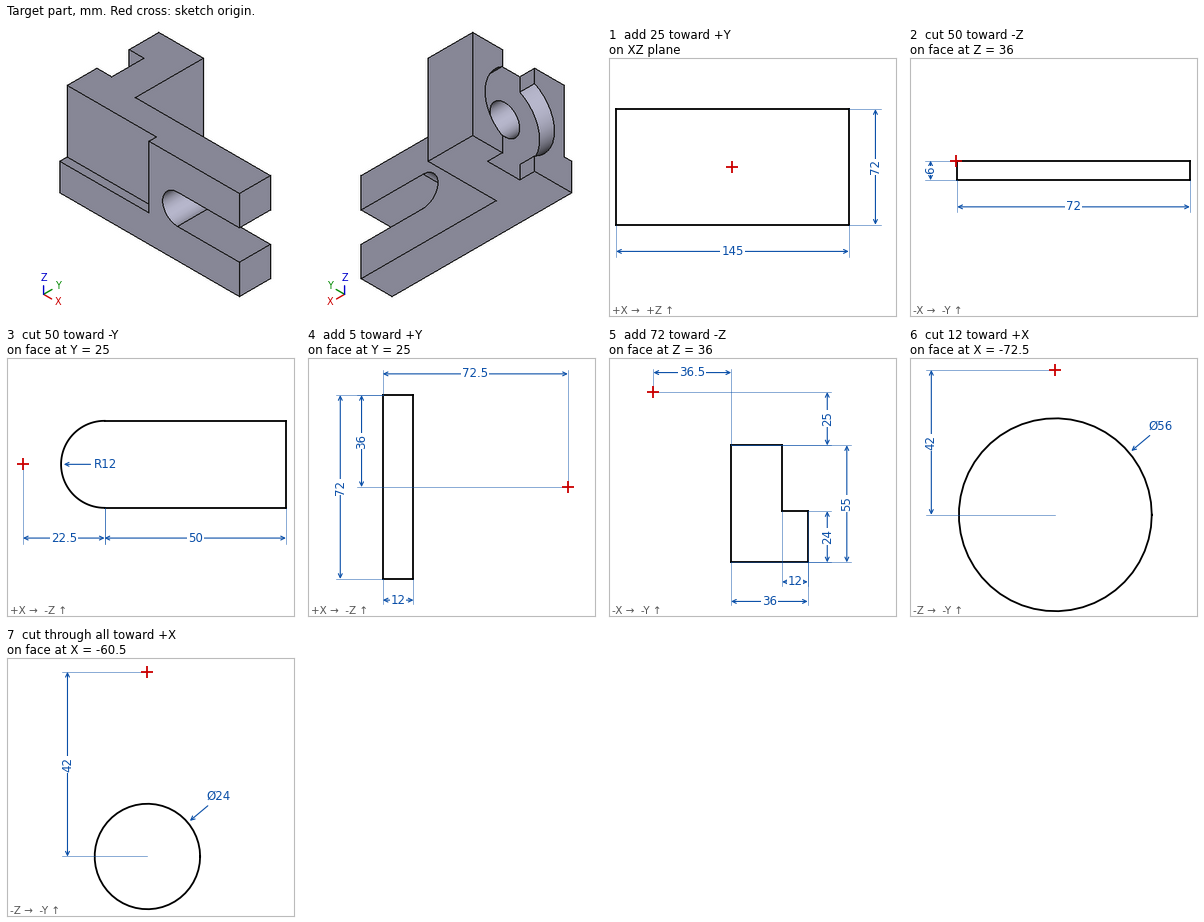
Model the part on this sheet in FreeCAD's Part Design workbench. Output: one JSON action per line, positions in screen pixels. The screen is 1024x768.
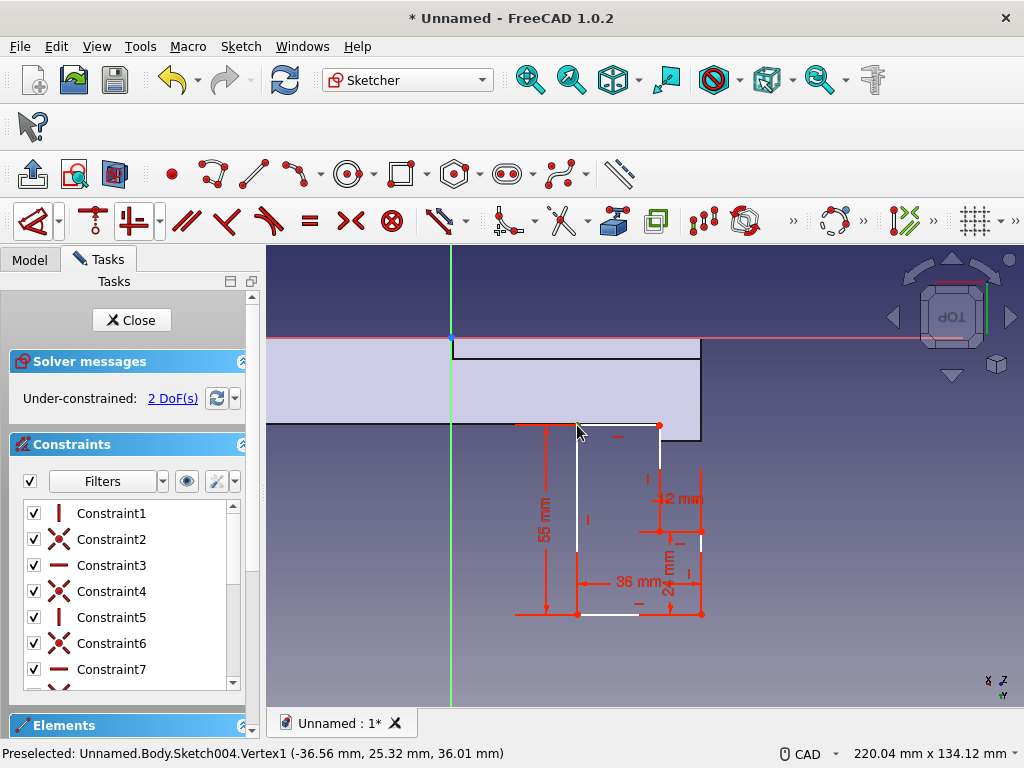
{"action": "left_click", "coordinate": [58, 222]}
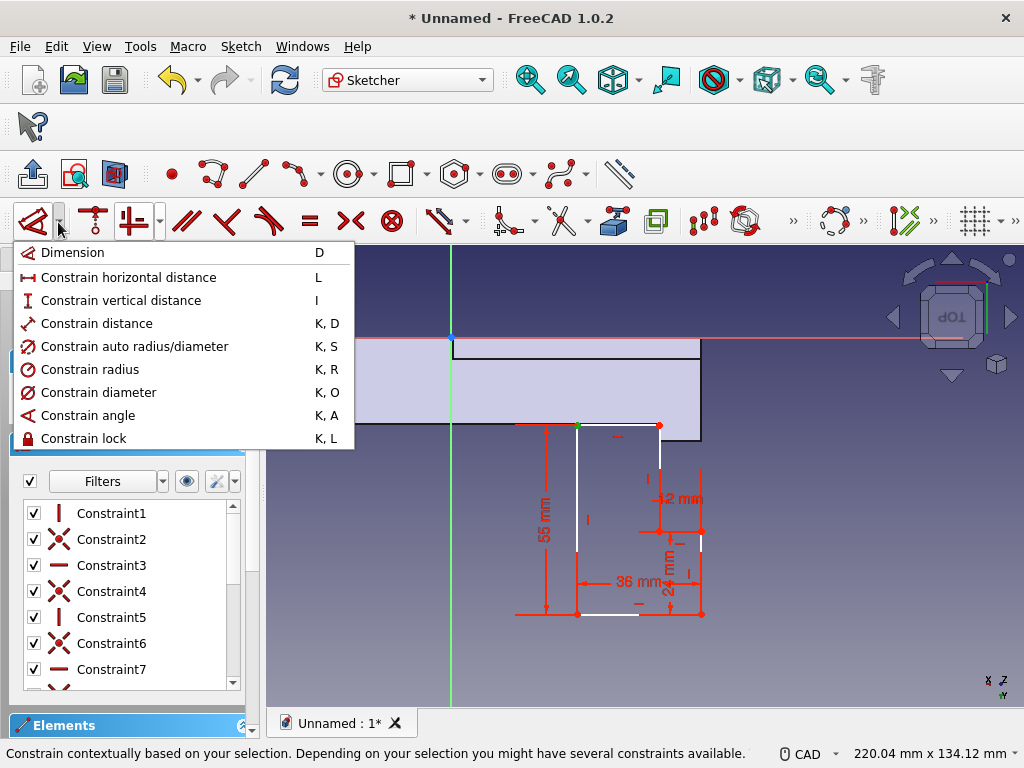
{"action": "left_click", "coordinate": [184, 300]}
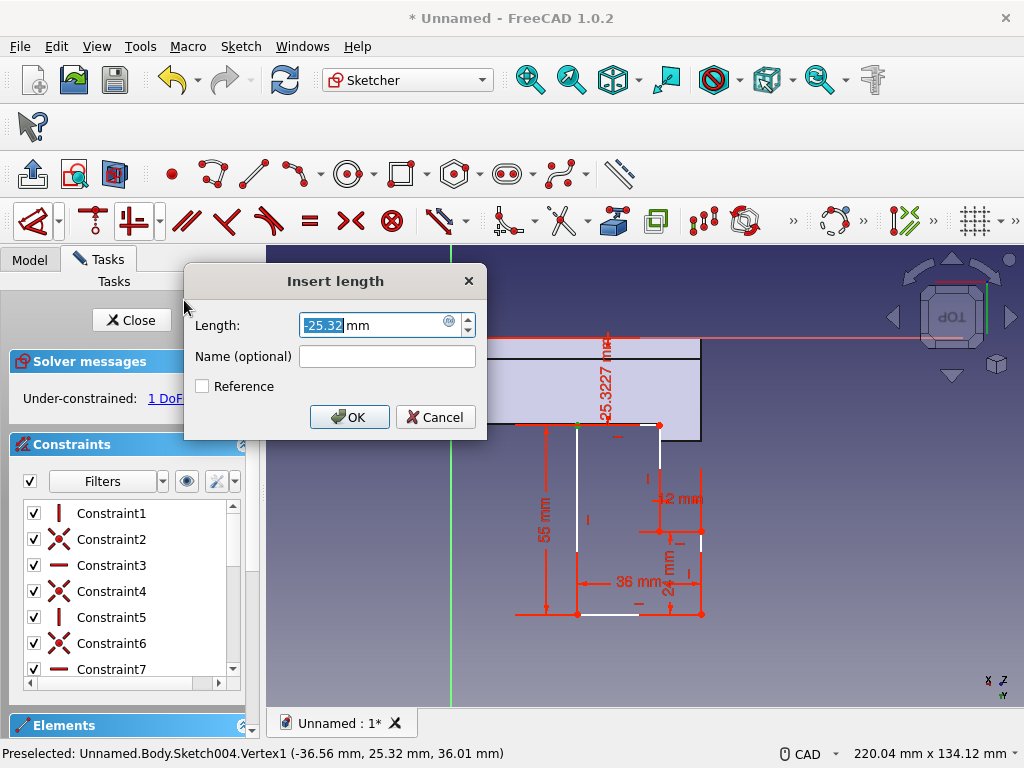
{"action": "type", "text": "-25"}
{"action": "key", "text": "Return"}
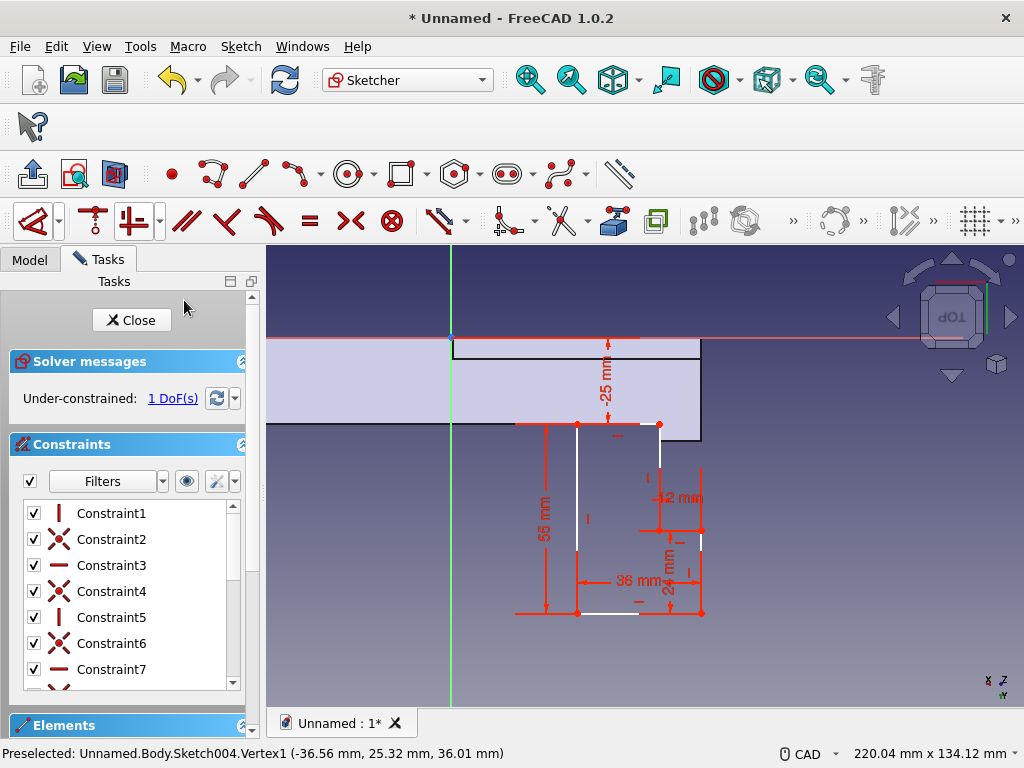
{"action": "left_click", "coordinate": [577, 424]}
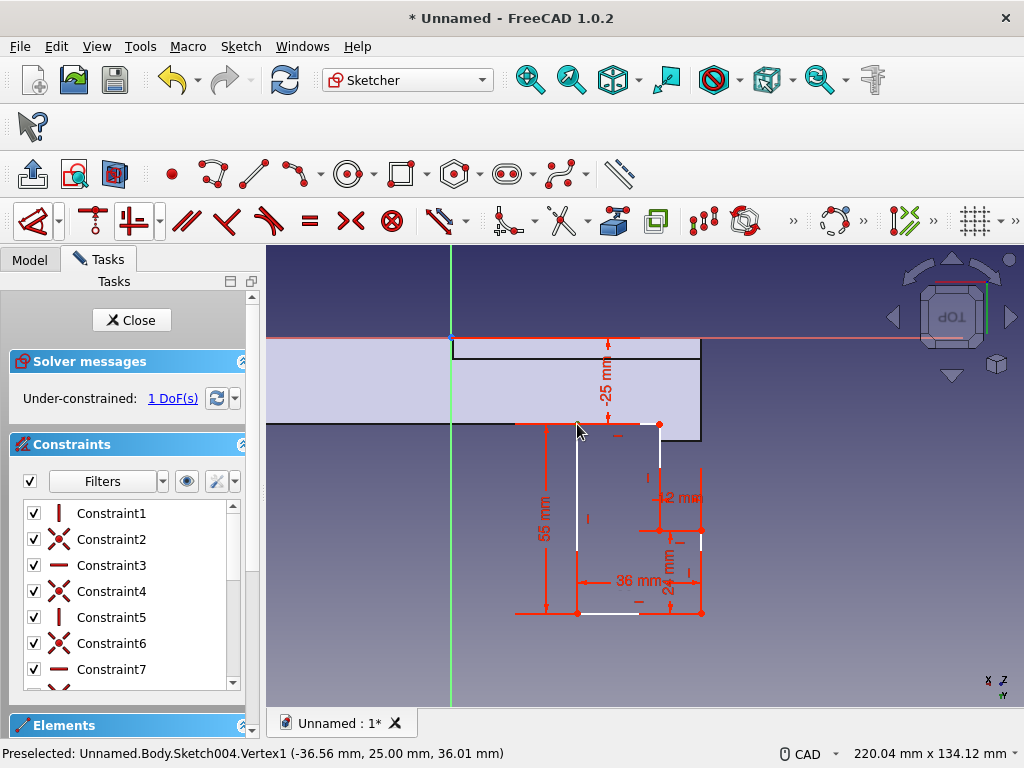
{"action": "left_click", "coordinate": [58, 222]}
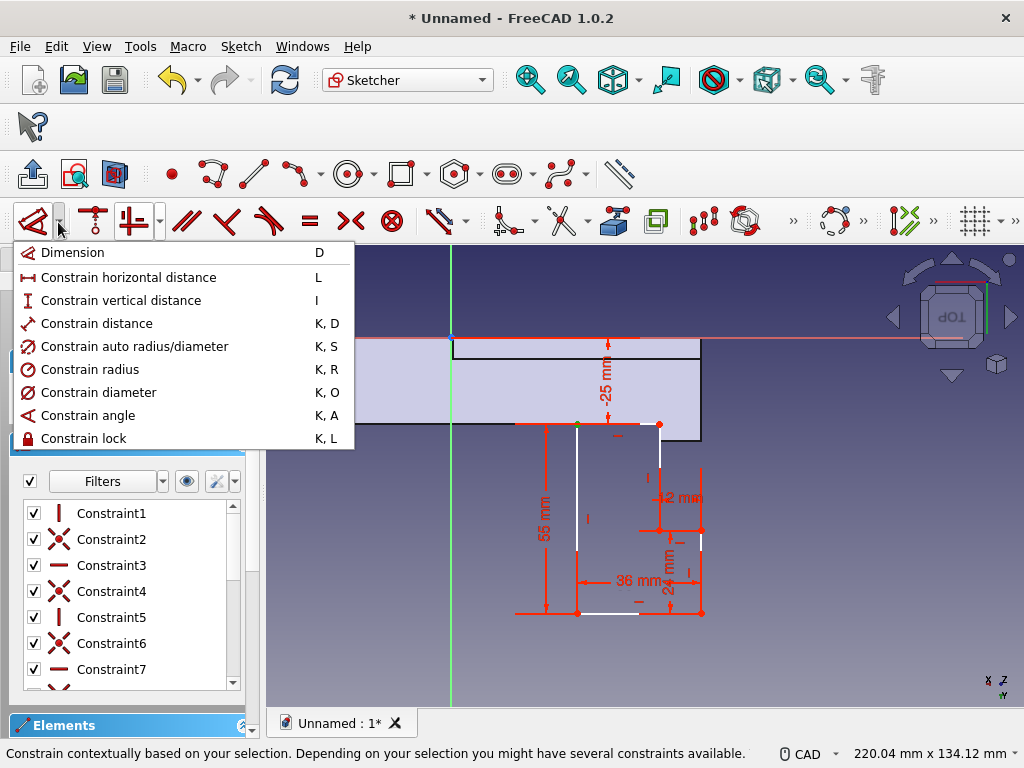
{"action": "left_click", "coordinate": [184, 278]}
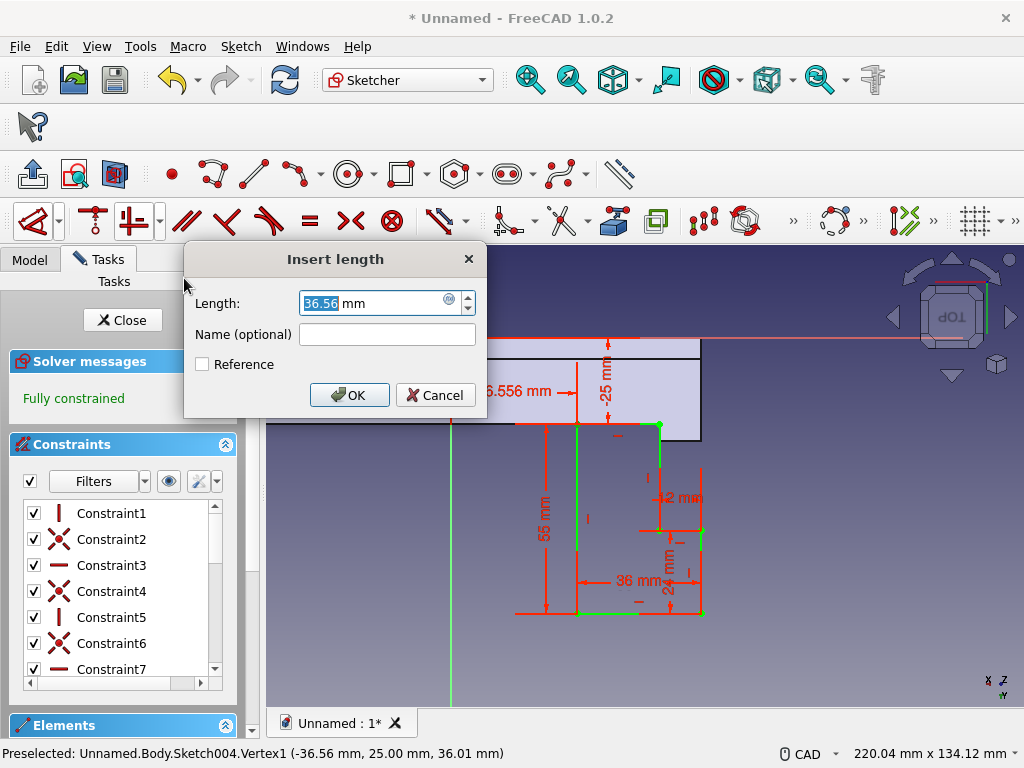
{"action": "type", "text": "36.5"}
{"action": "key", "text": "Return"}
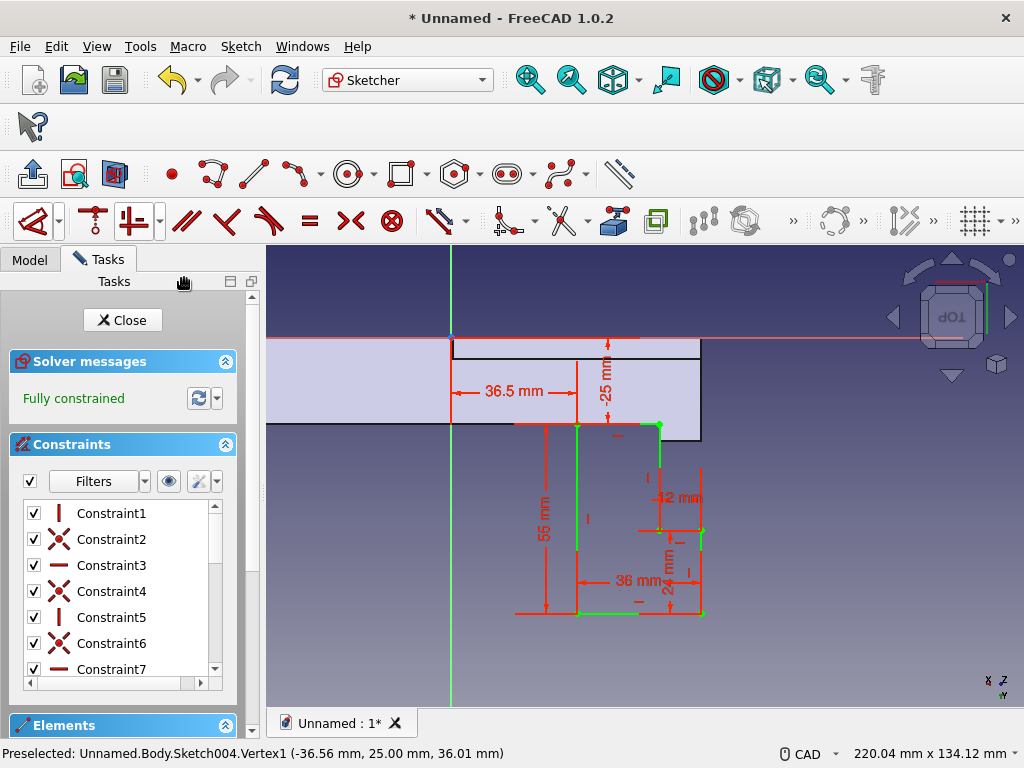
{"action": "left_click", "coordinate": [123, 320]}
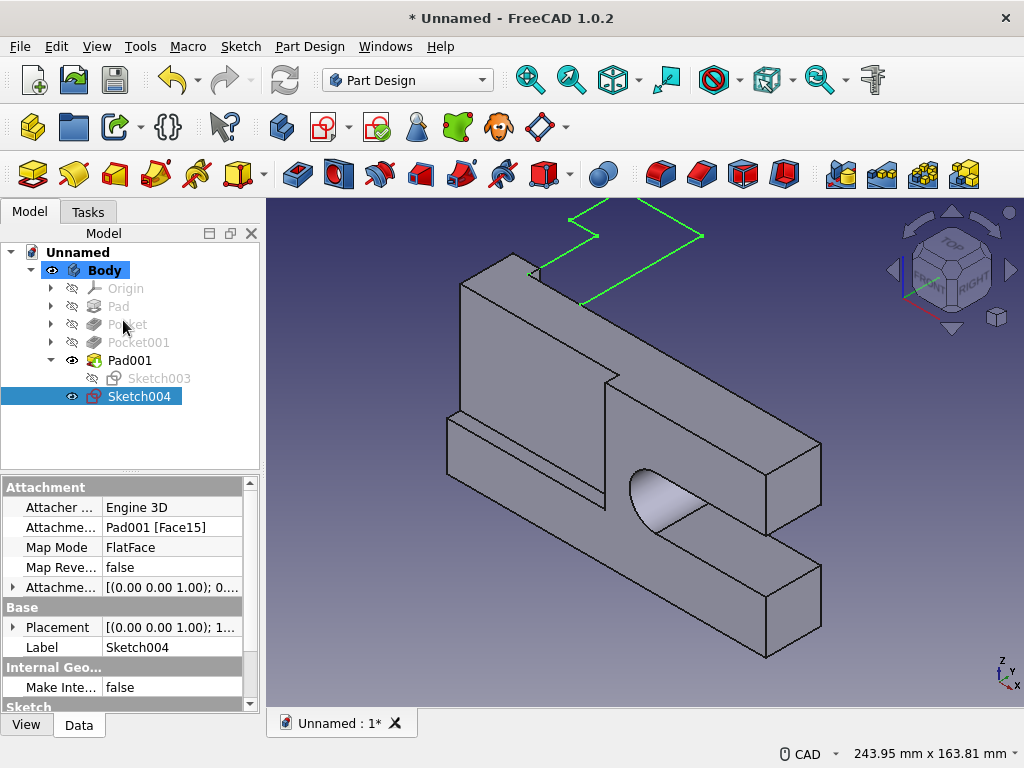
{"action": "left_click", "coordinate": [33, 174]}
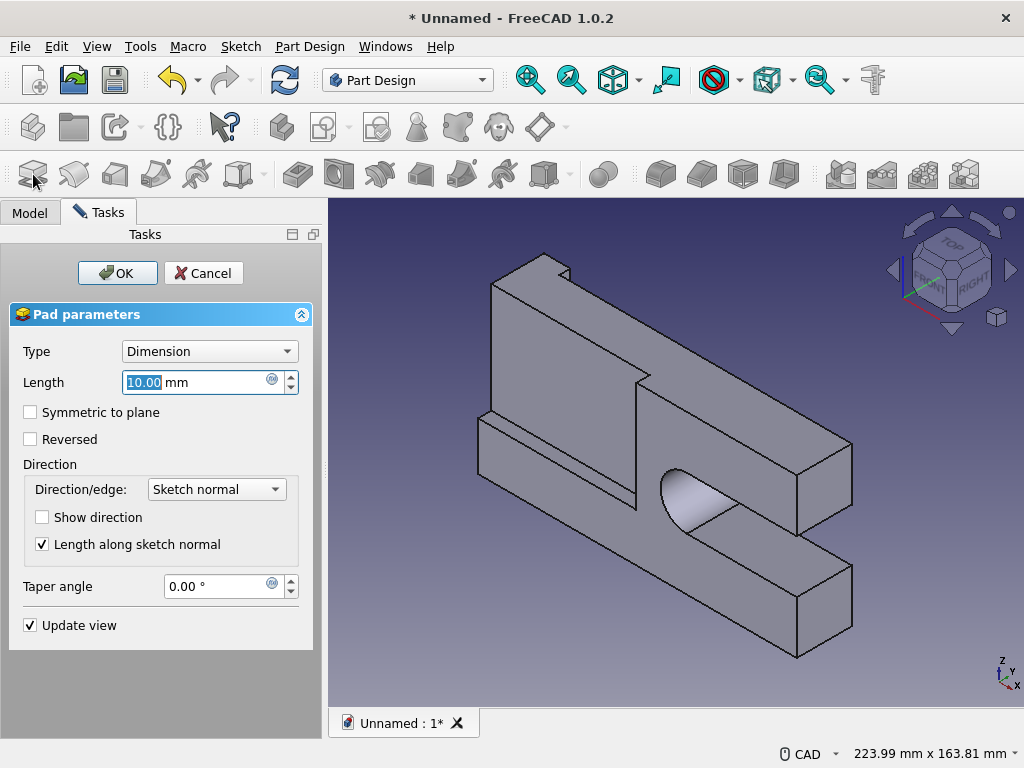
{"action": "type", "text": "72"}
{"action": "key", "text": "Tab"}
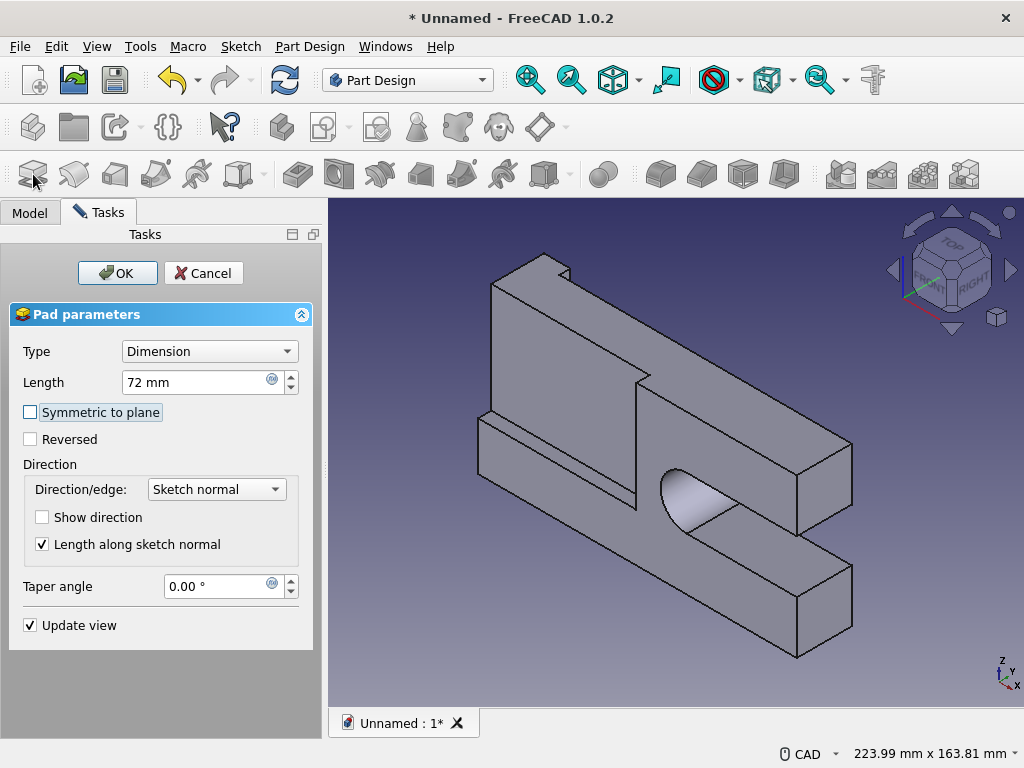
{"action": "left_click", "coordinate": [31, 439]}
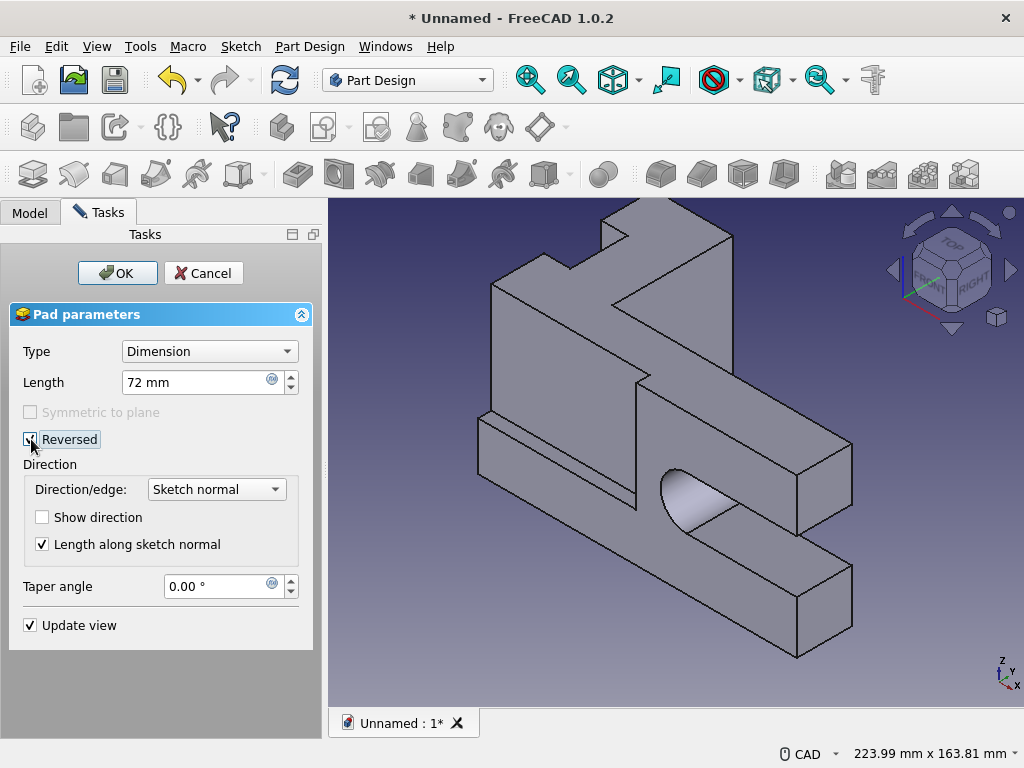
{"action": "left_click", "coordinate": [118, 273]}